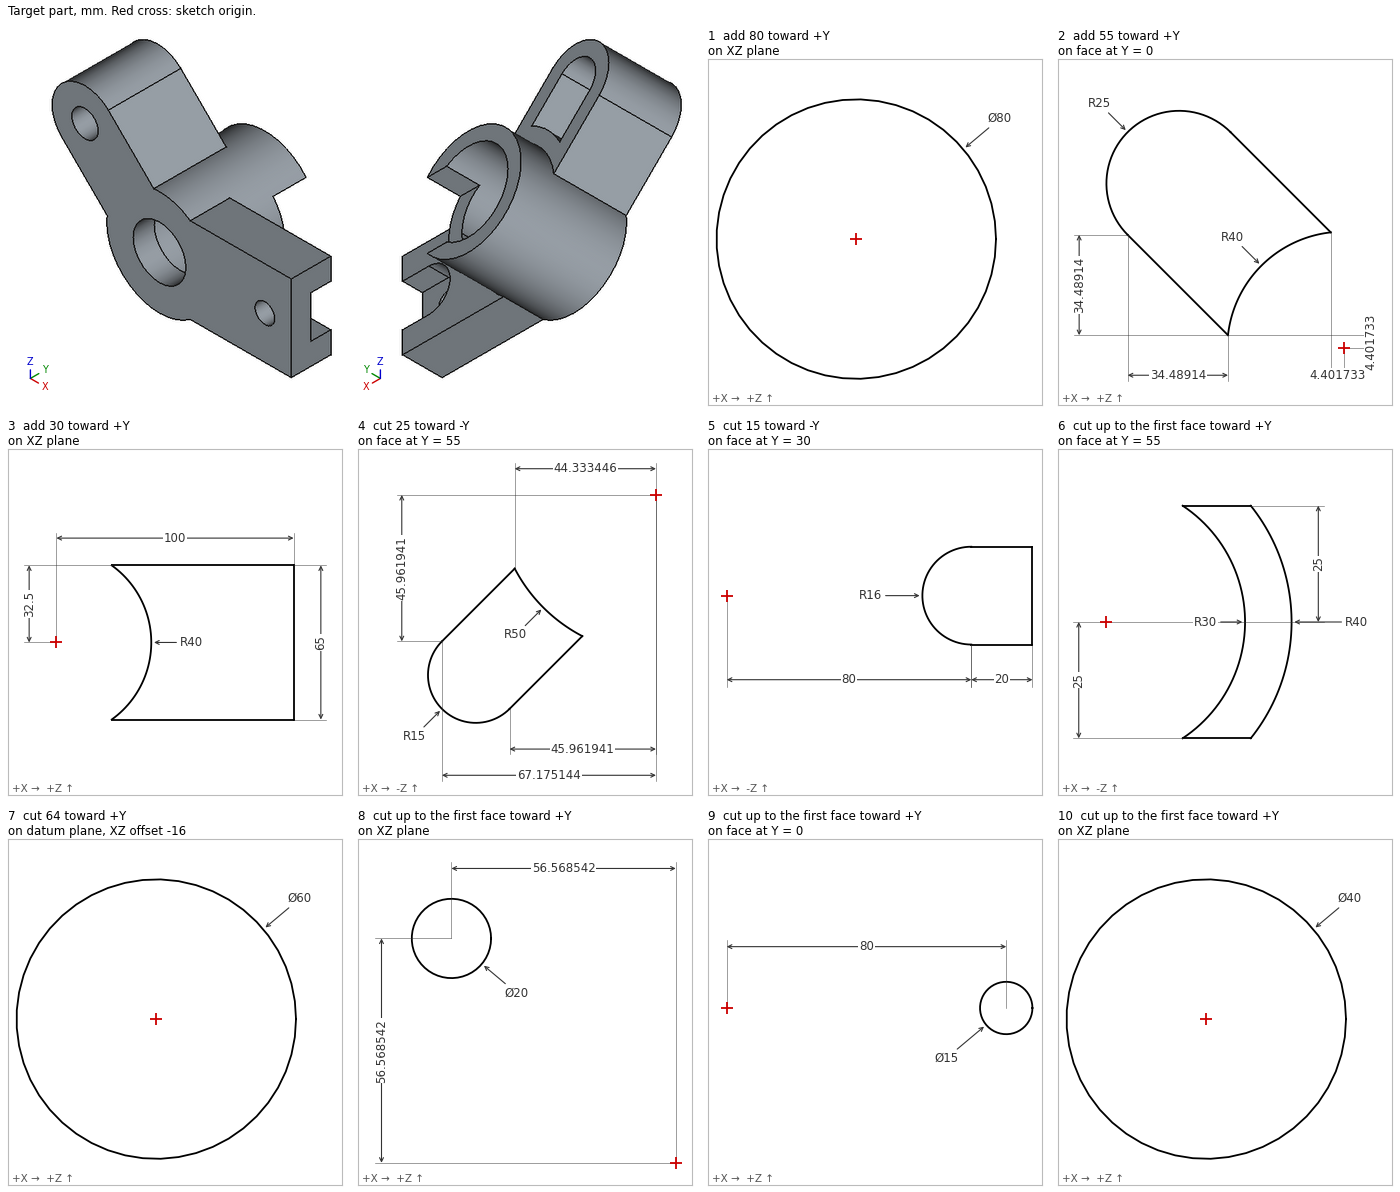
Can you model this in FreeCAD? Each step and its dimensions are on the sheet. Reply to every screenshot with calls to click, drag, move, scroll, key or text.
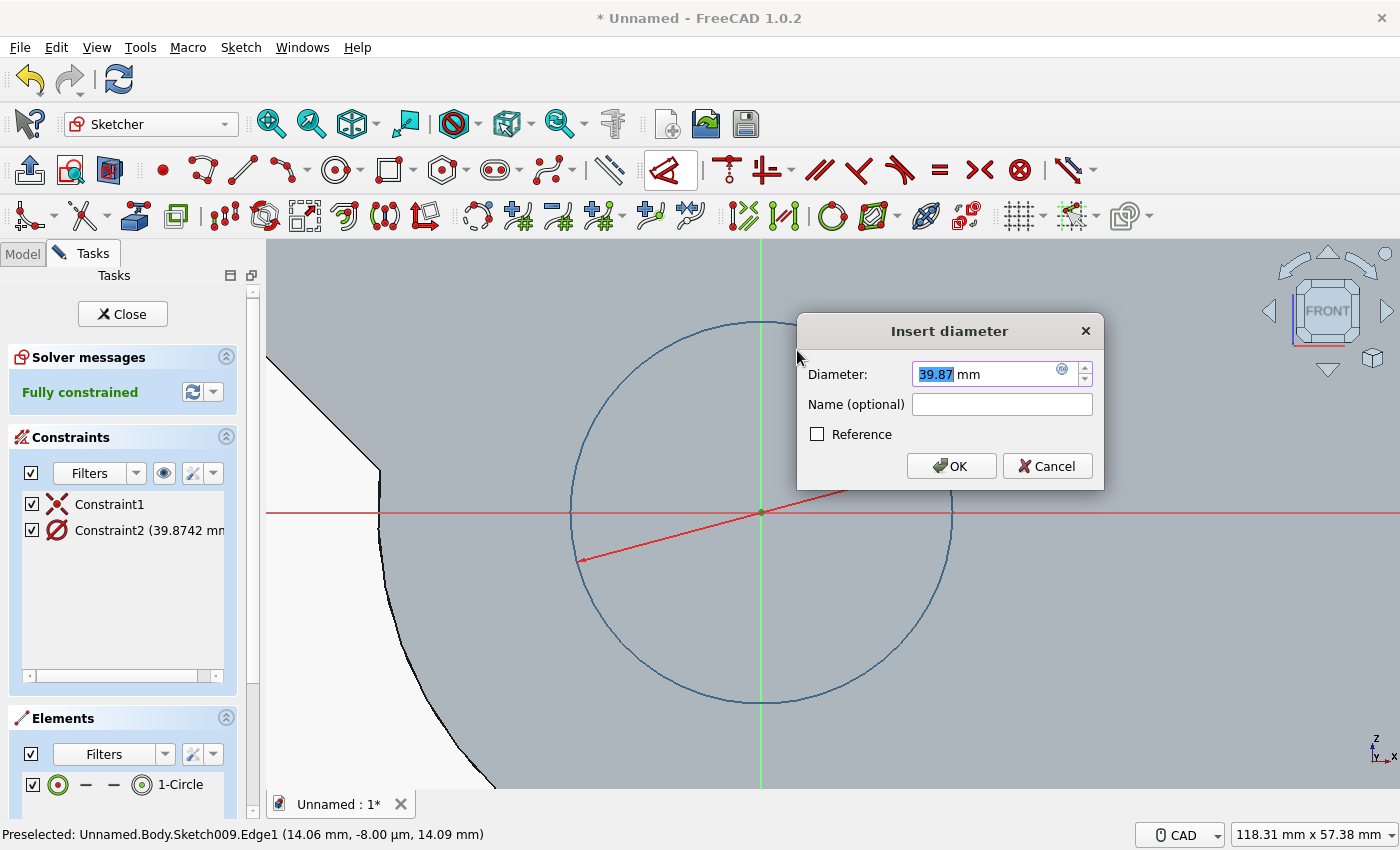
text(40)
key(Return)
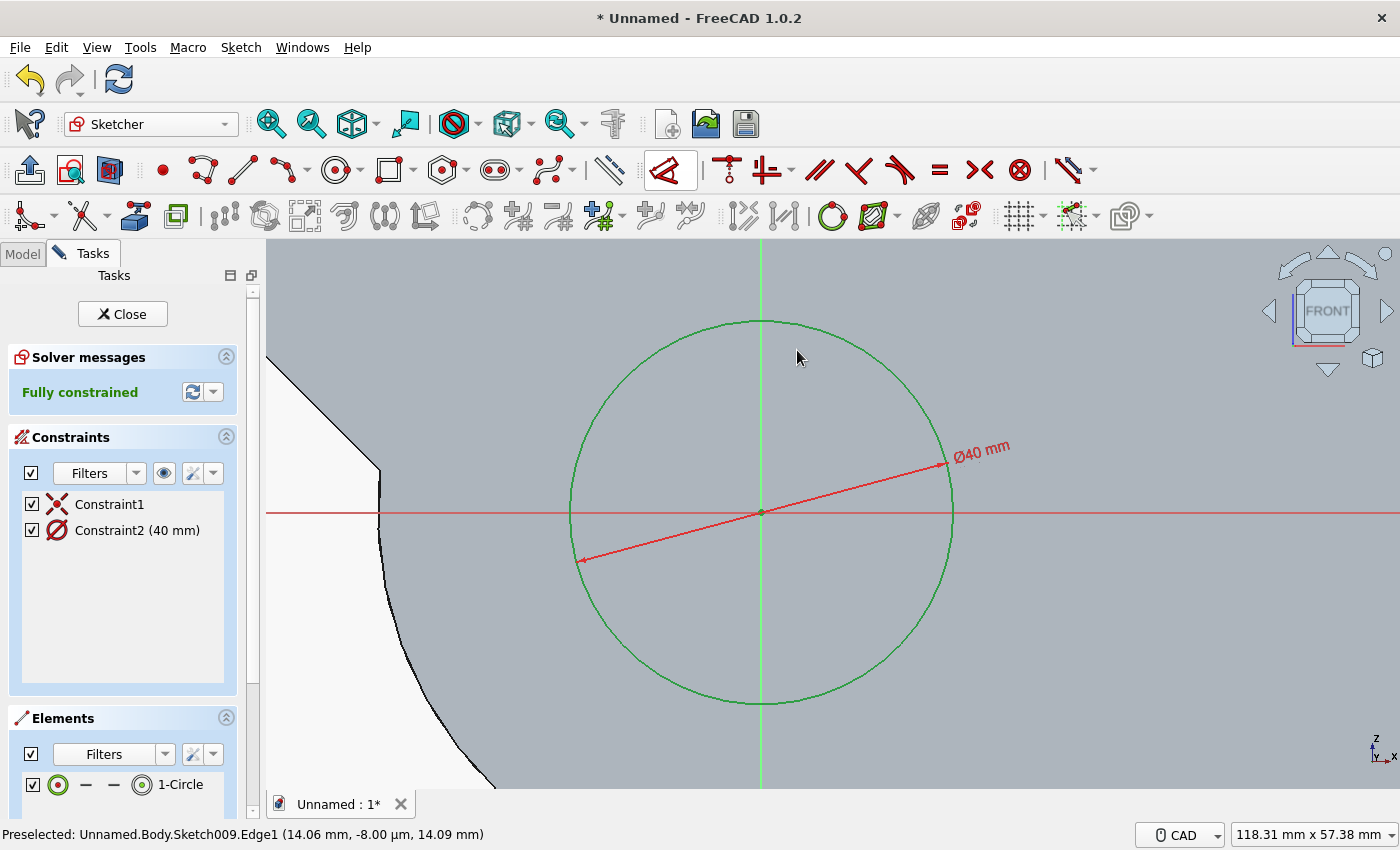
click(123, 314)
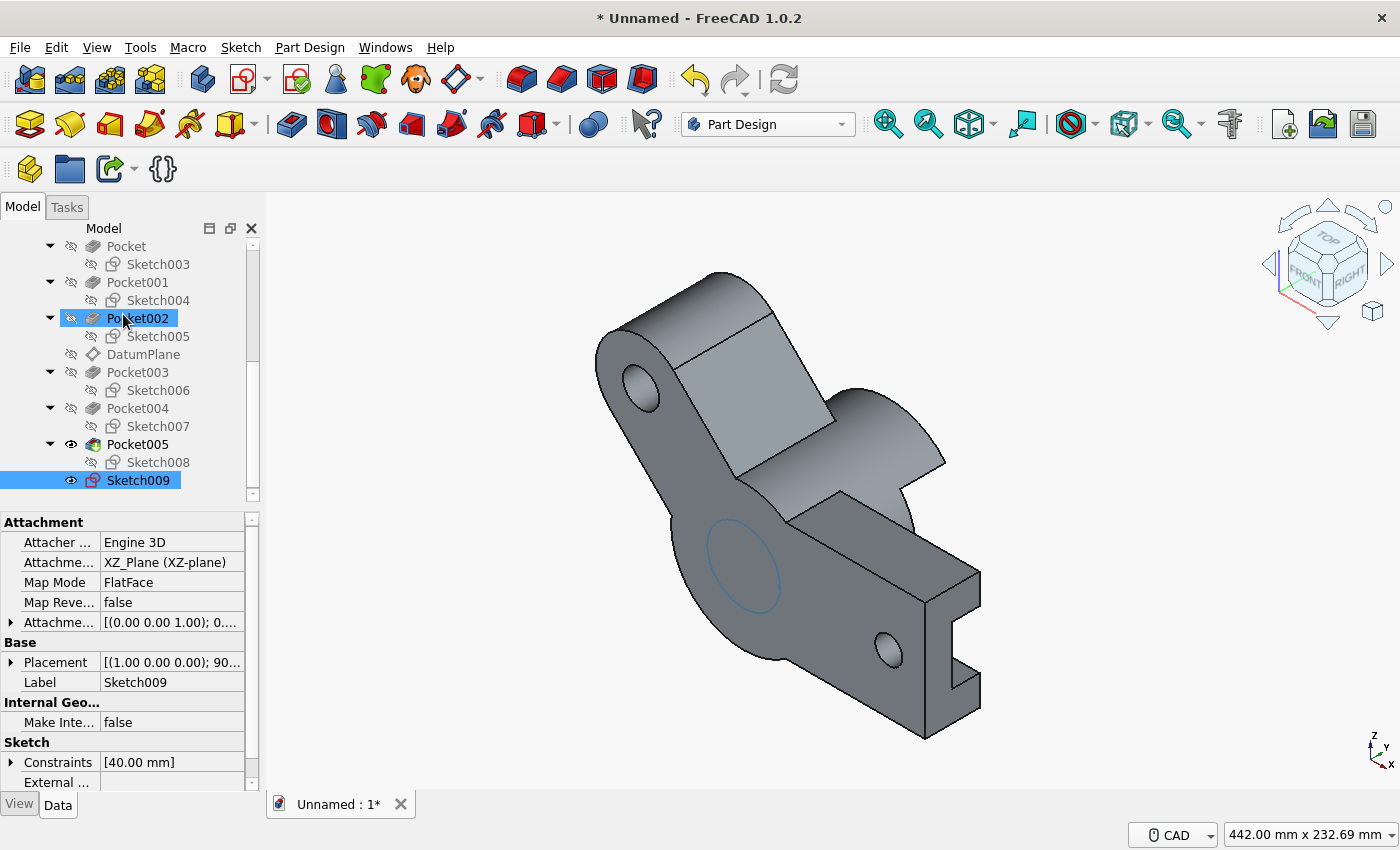
click(292, 124)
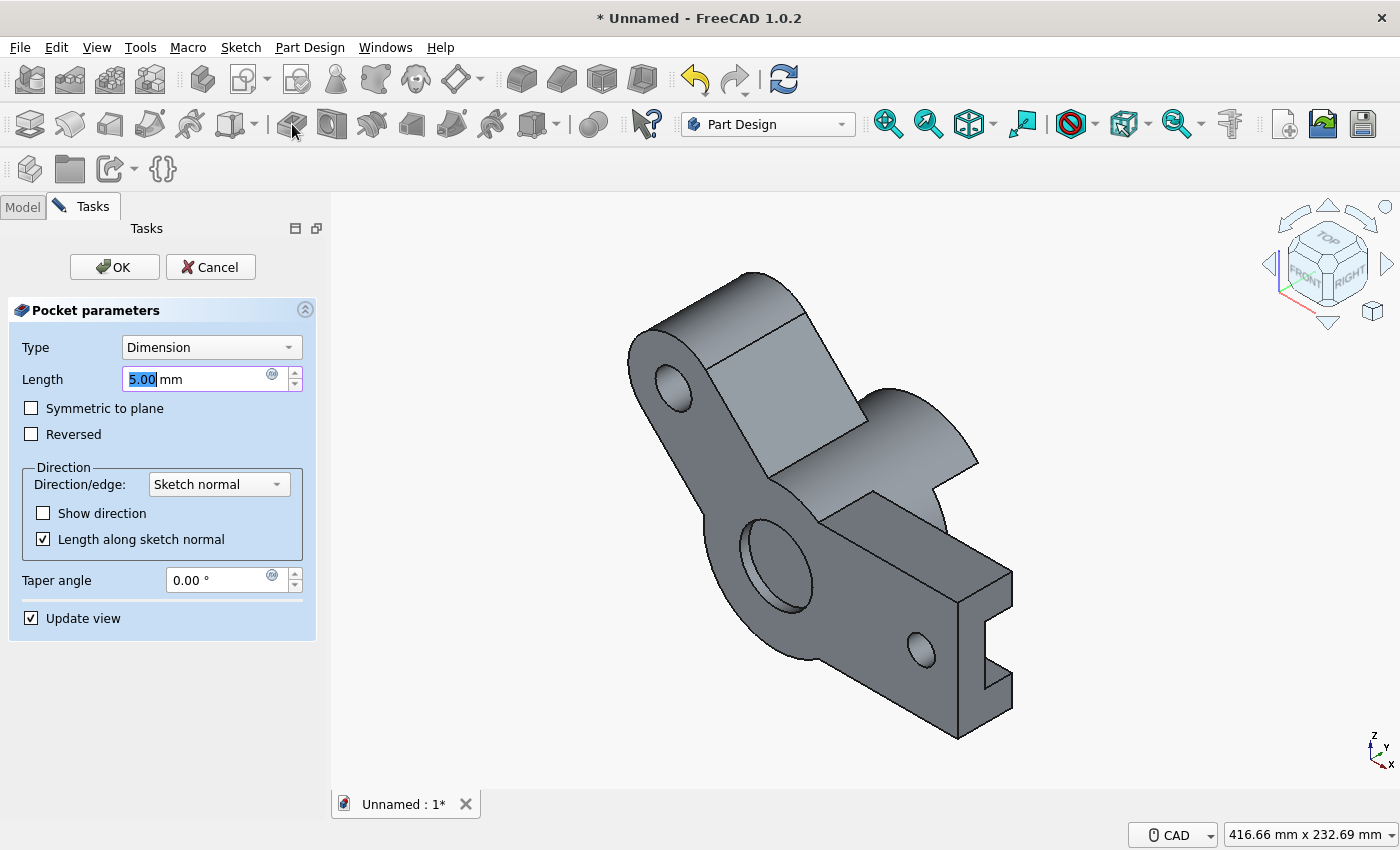
click(212, 348)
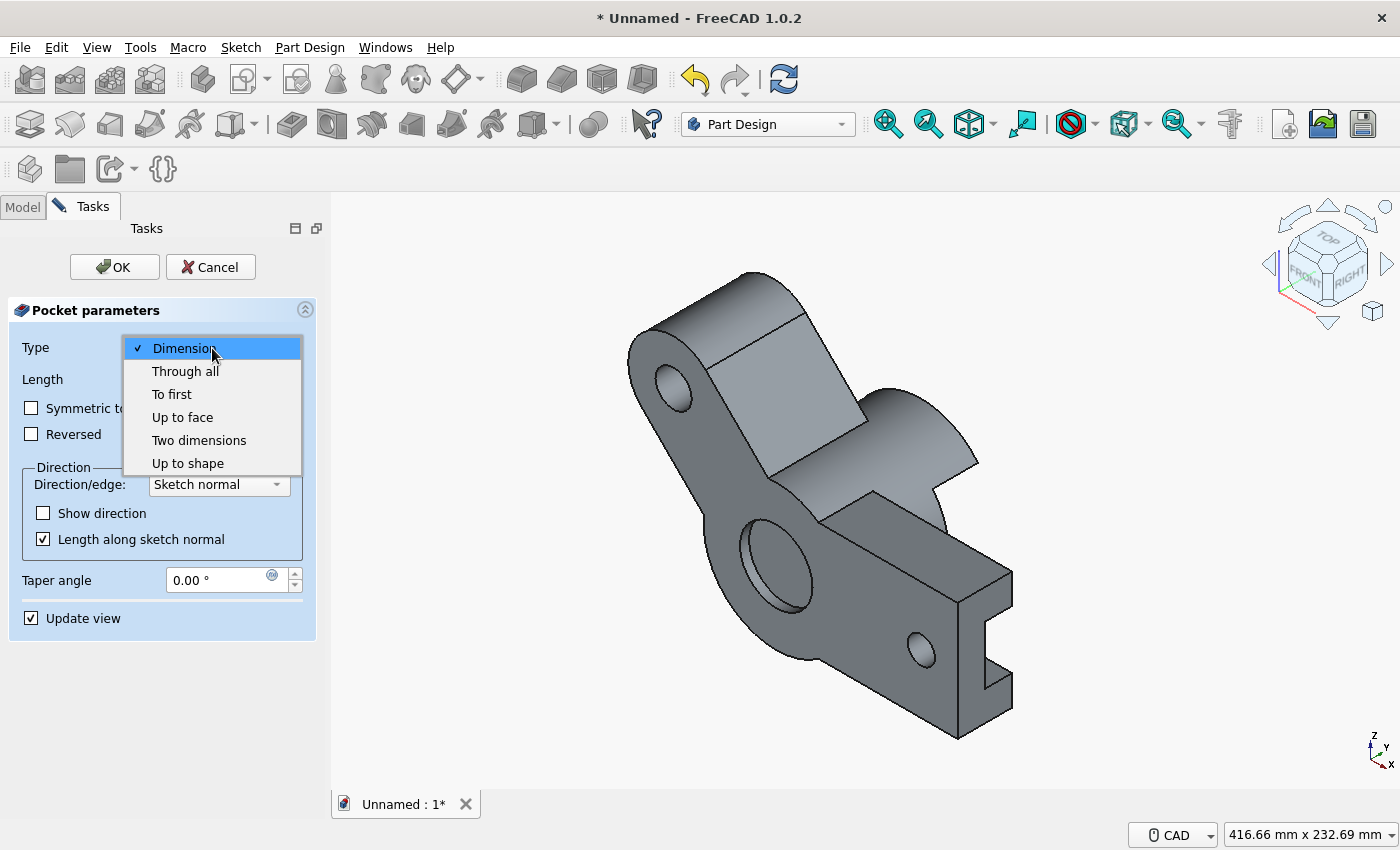
click(212, 394)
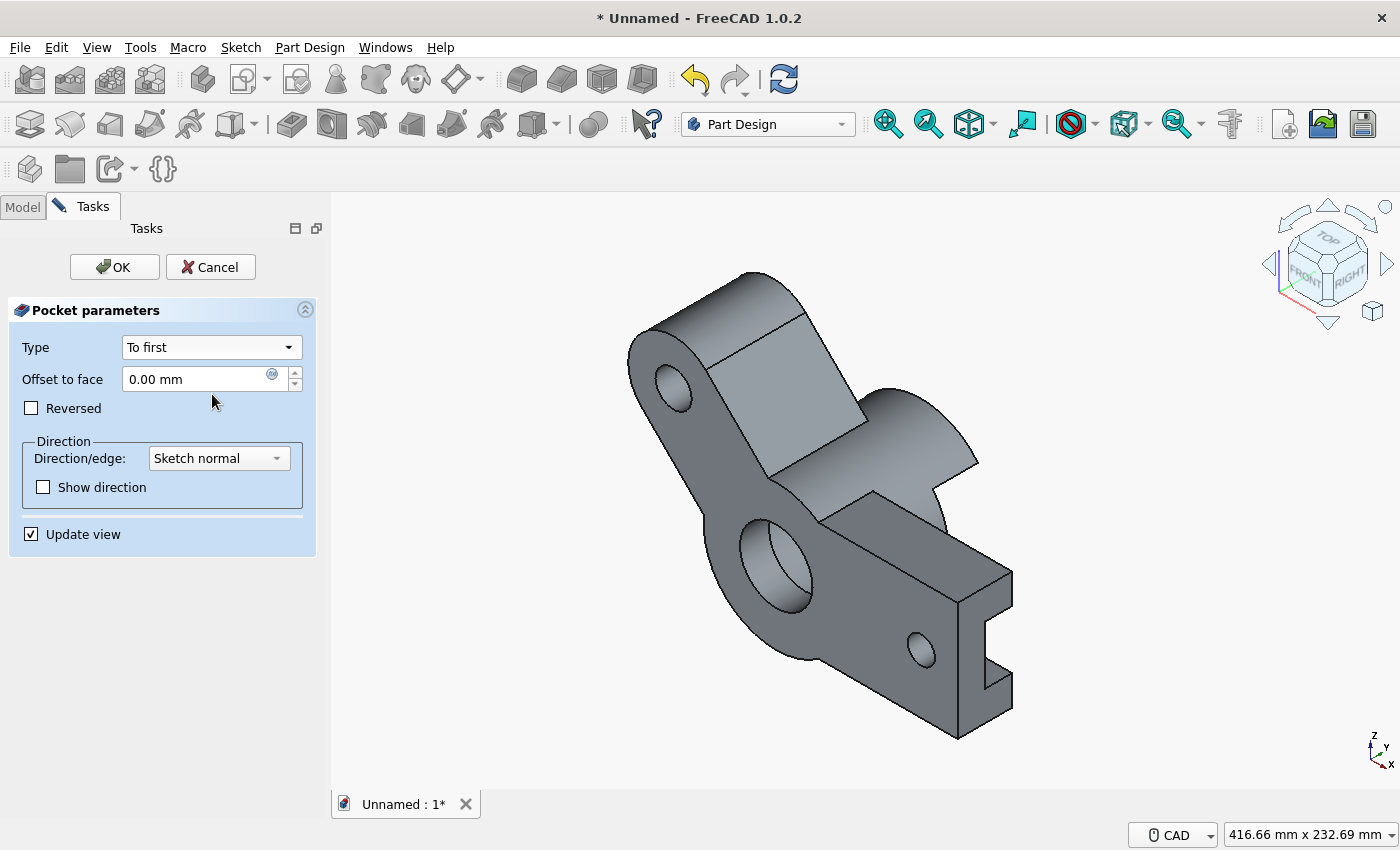
click(115, 267)